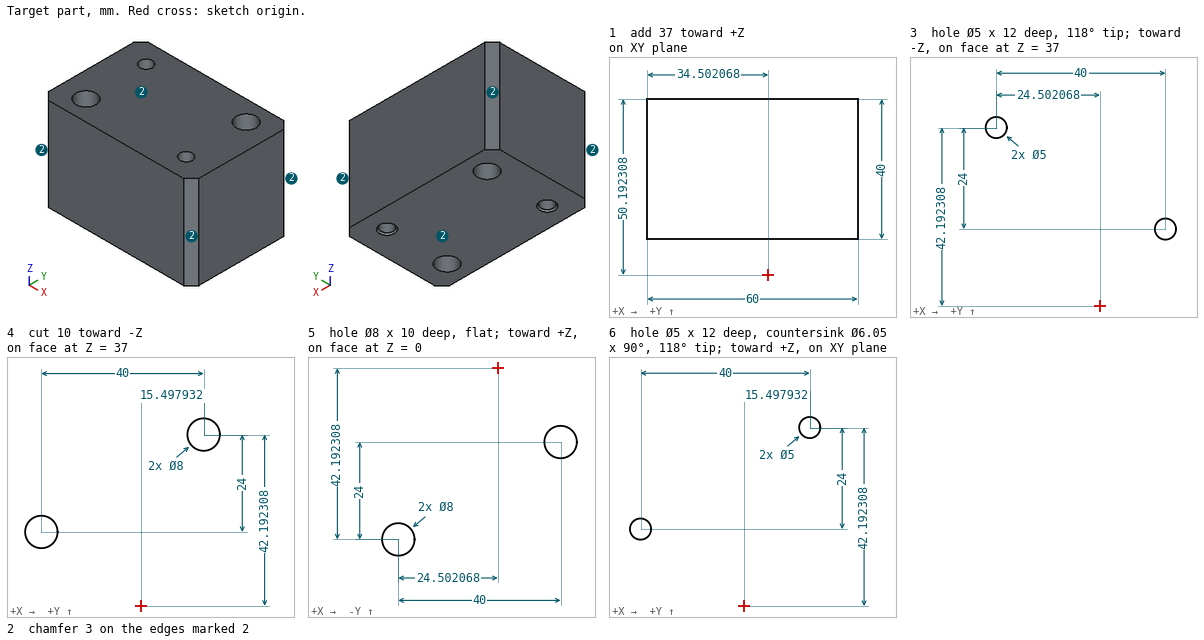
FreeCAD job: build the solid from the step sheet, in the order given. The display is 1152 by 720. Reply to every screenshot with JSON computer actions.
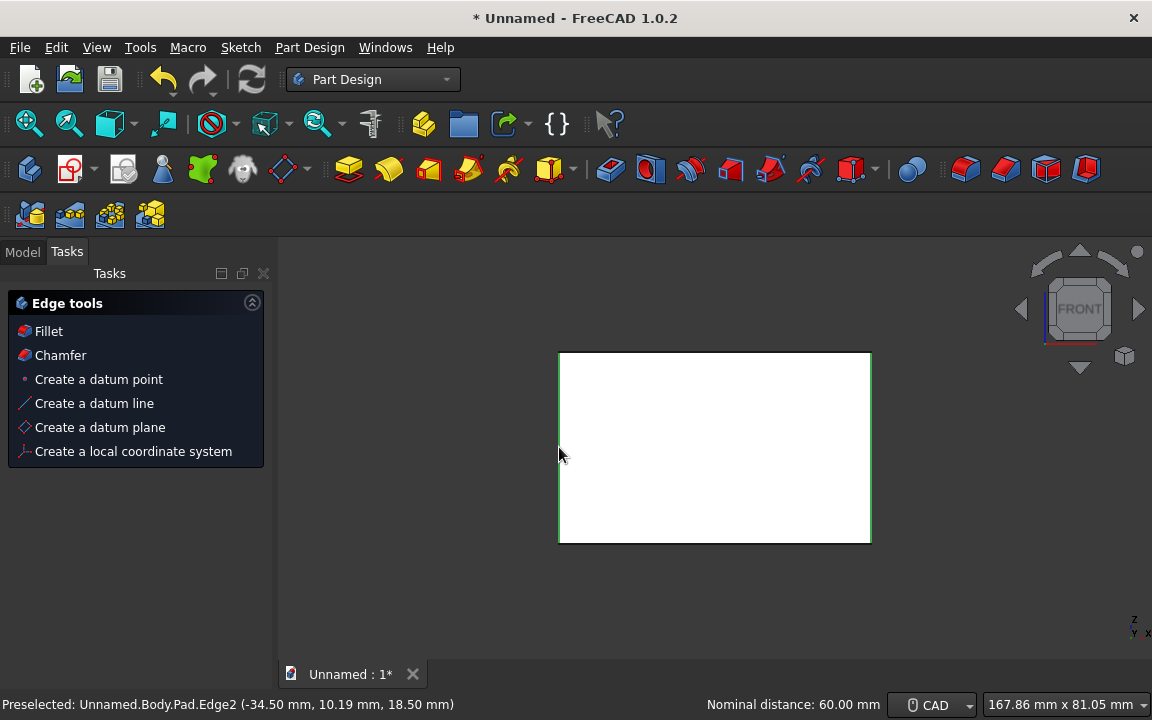
{"action": "key", "text": "3"}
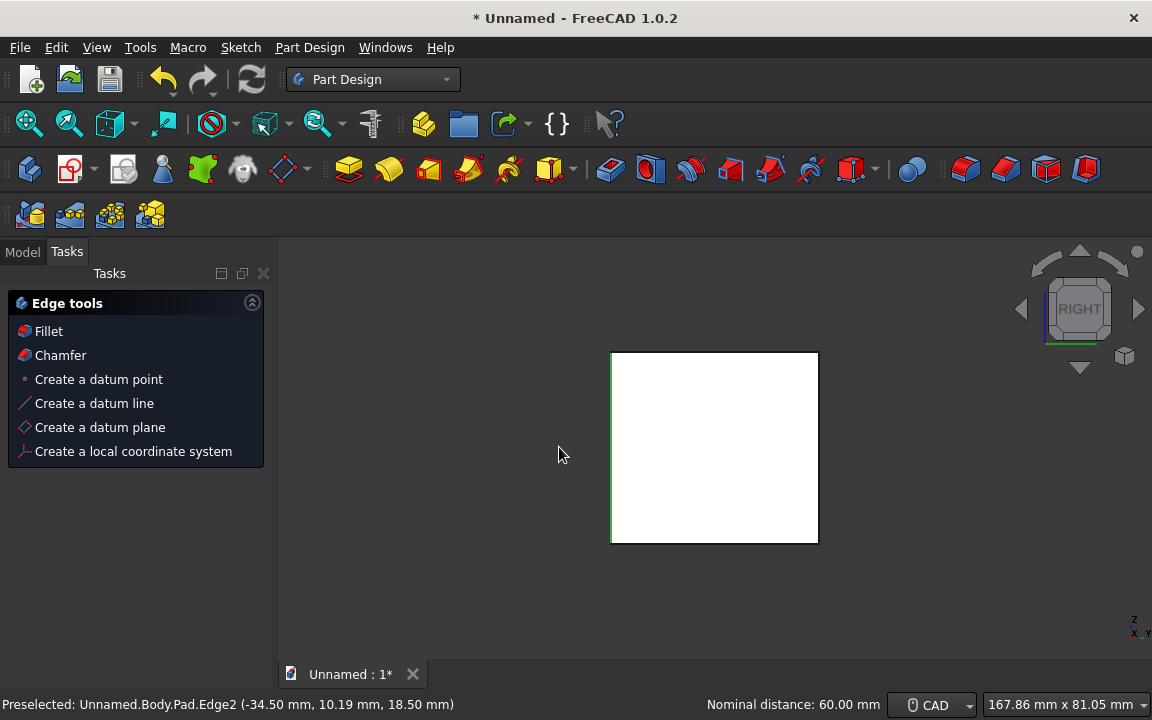
{"action": "left_click", "coordinate": [819, 447], "text": "ctrl"}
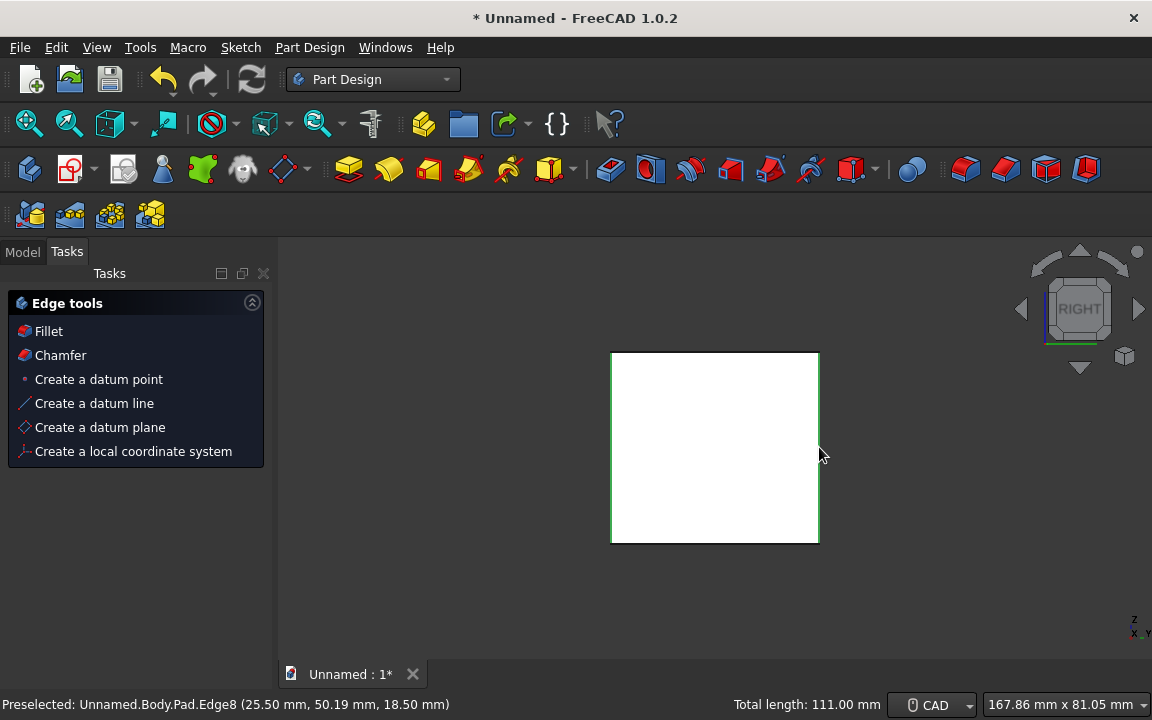
{"action": "key", "text": "5"}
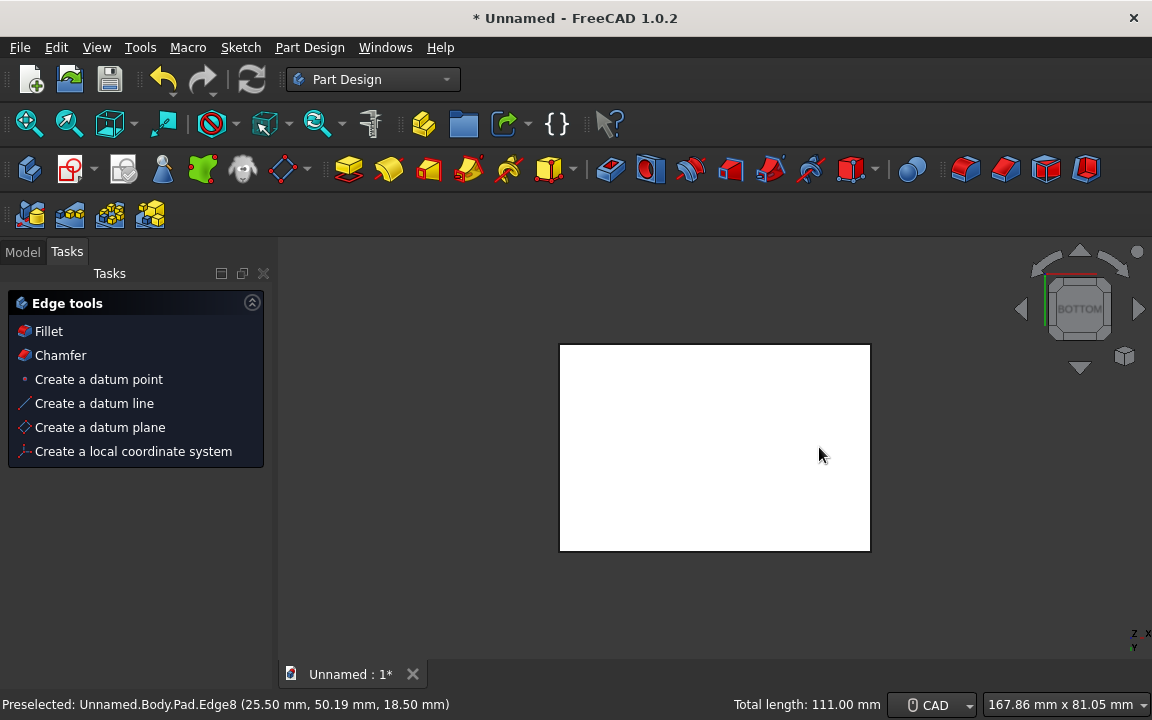
{"action": "key", "text": "4"}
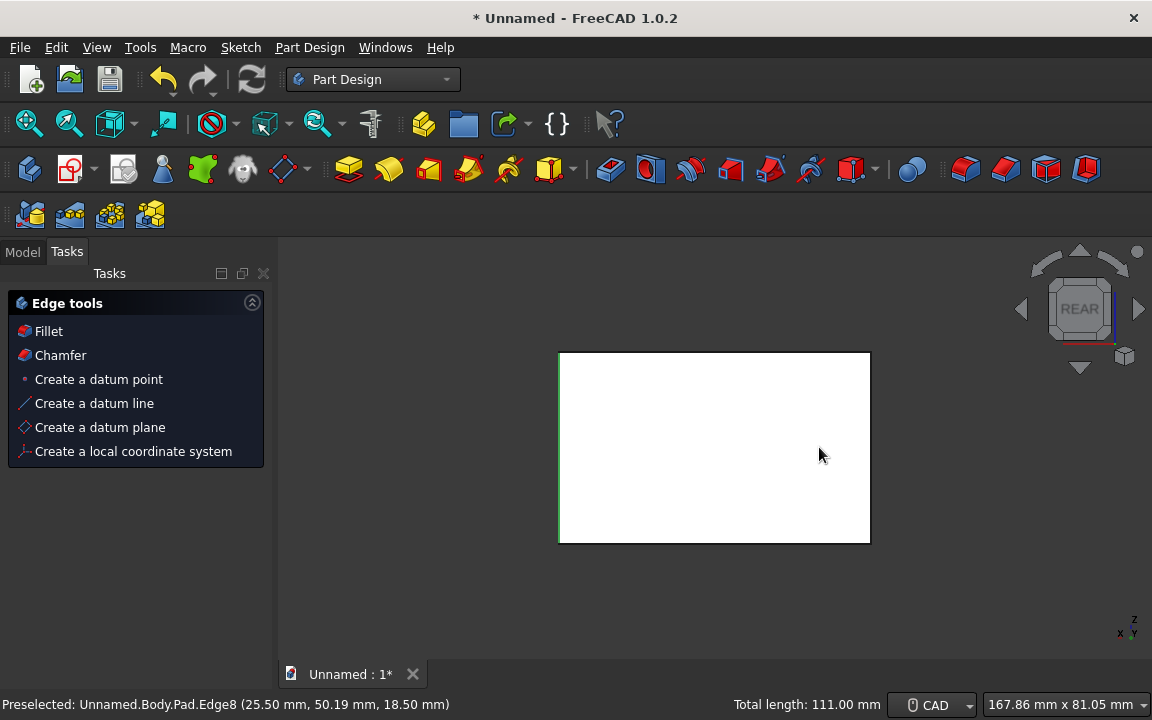
{"action": "left_click", "coordinate": [871, 447], "text": "ctrl"}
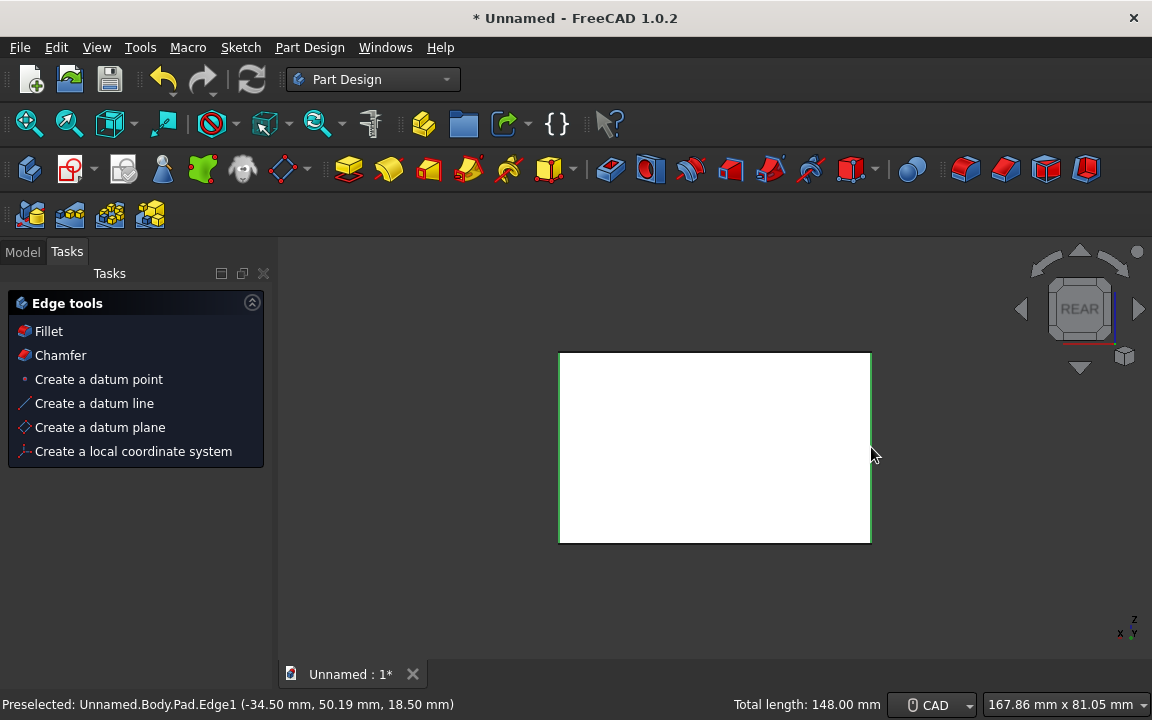
{"action": "left_click", "coordinate": [1006, 170]}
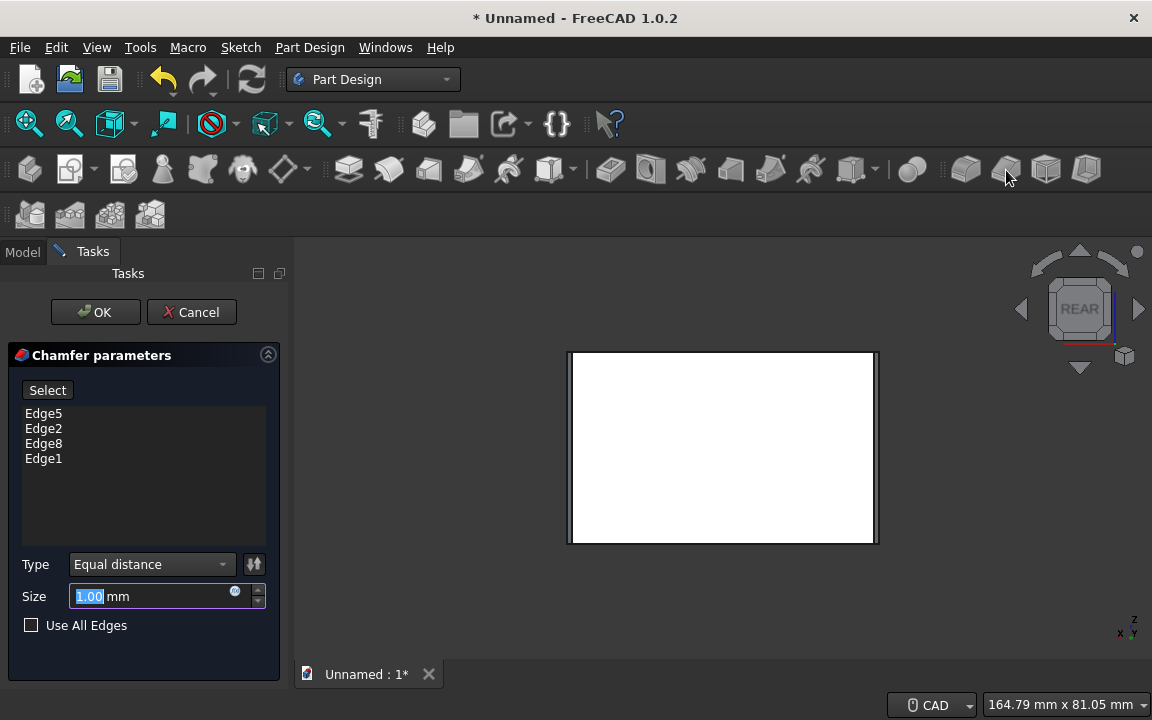
{"action": "type", "text": "3"}
{"action": "key", "text": "Tab"}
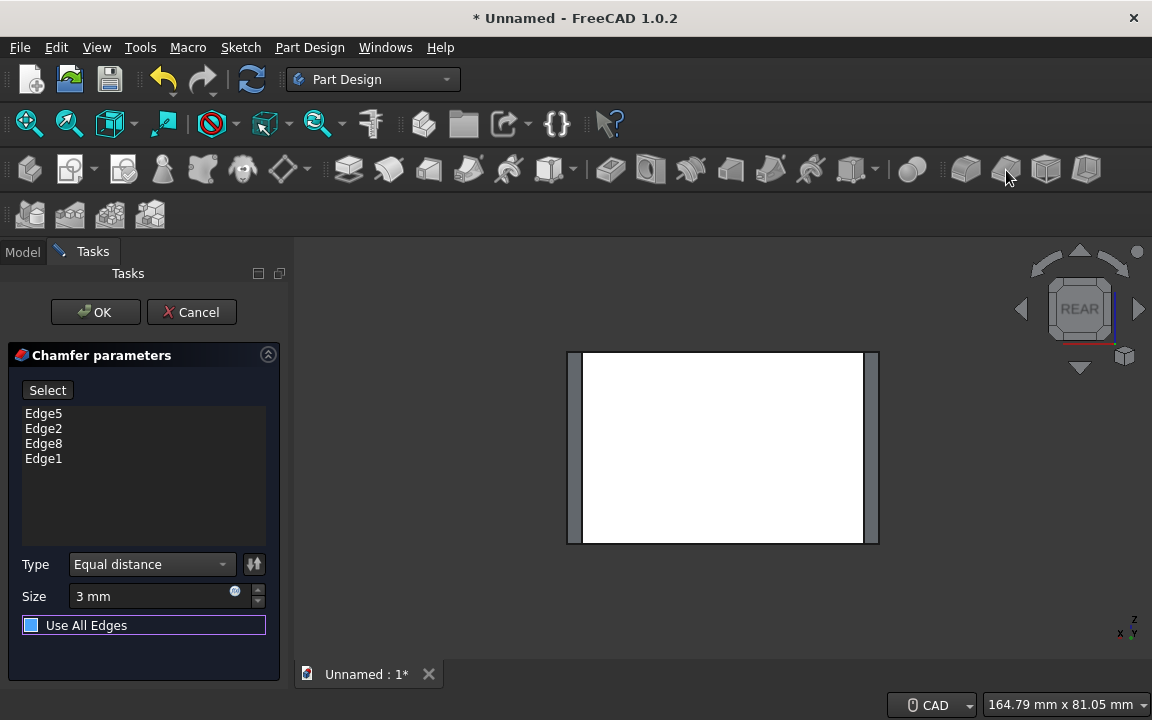
{"action": "left_click", "coordinate": [96, 312]}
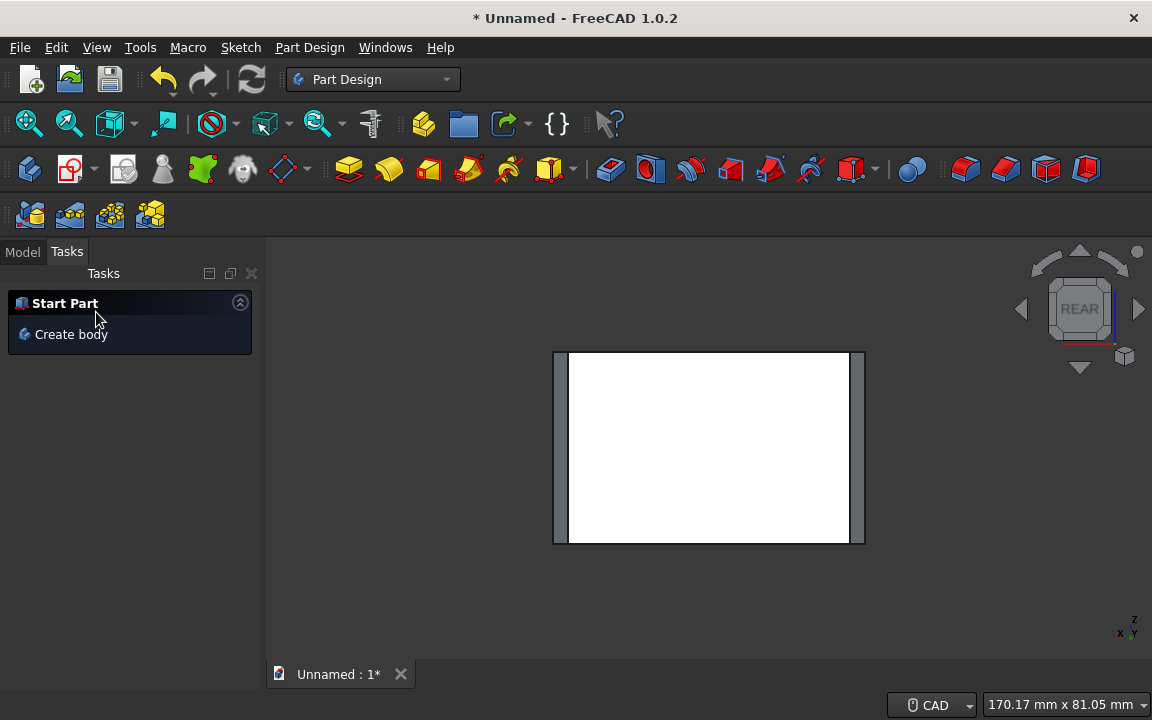
{"action": "key", "text": "0"}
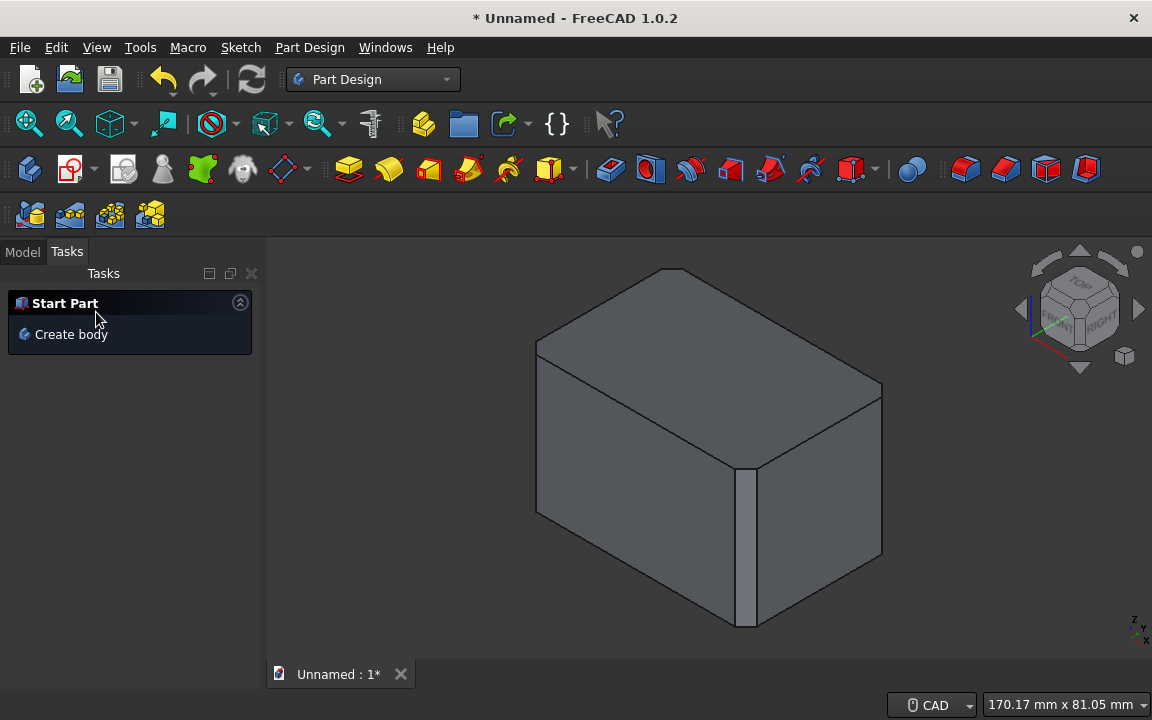
{"action": "left_click", "coordinate": [741, 387]}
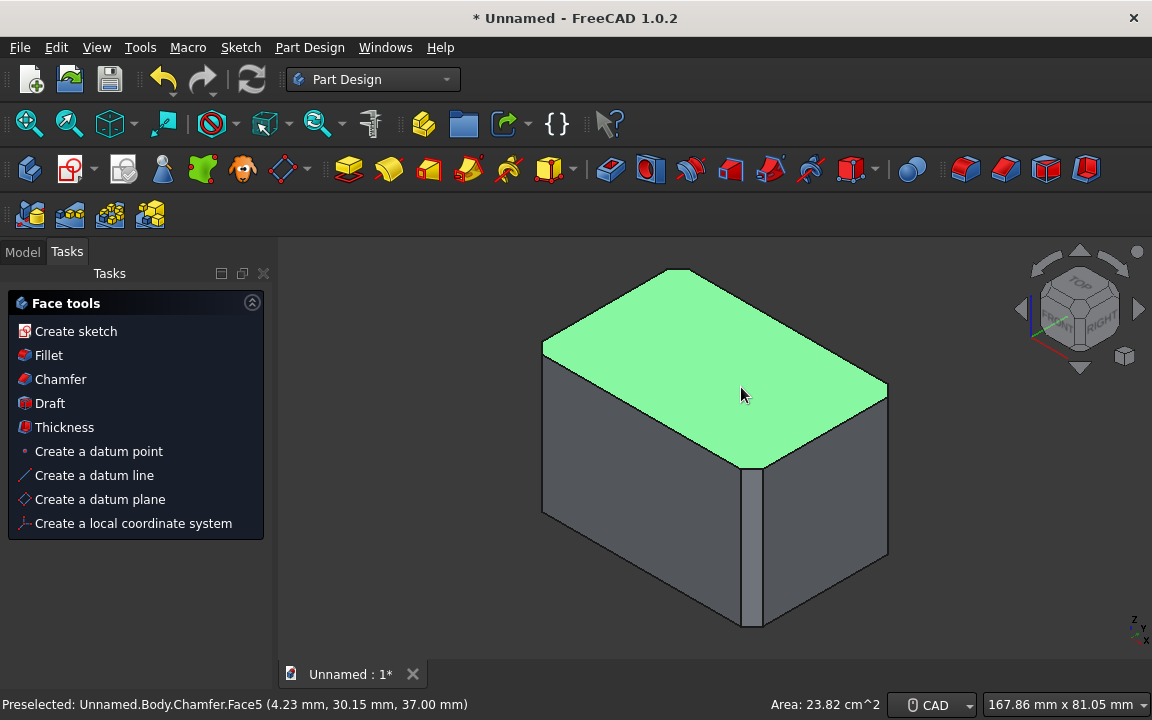
{"action": "left_click", "coordinate": [70, 170]}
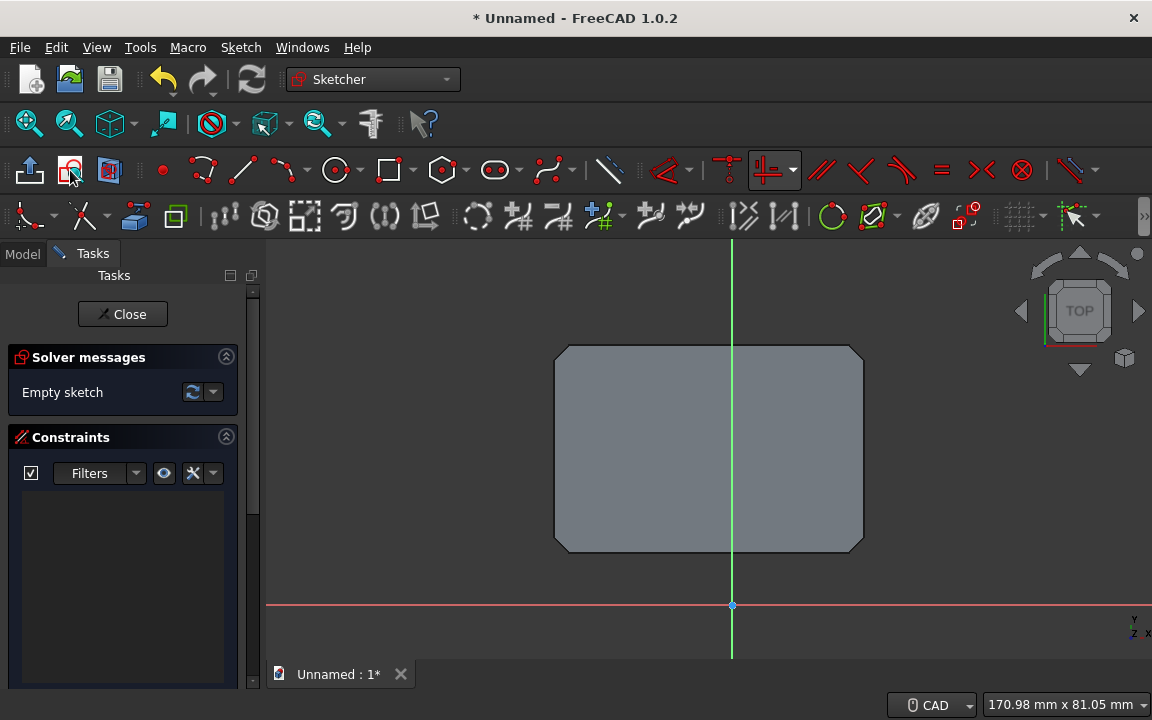
{"action": "left_click", "coordinate": [336, 170]}